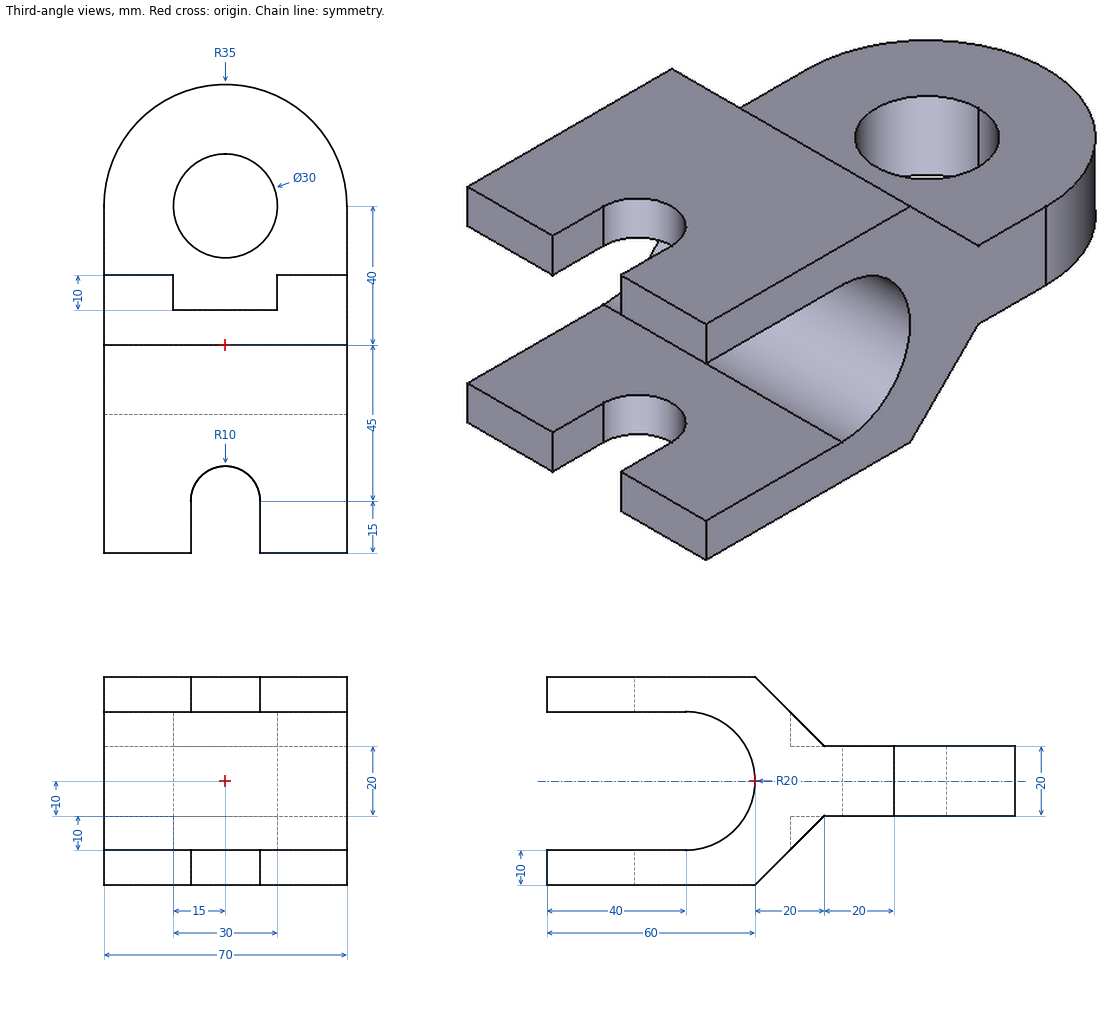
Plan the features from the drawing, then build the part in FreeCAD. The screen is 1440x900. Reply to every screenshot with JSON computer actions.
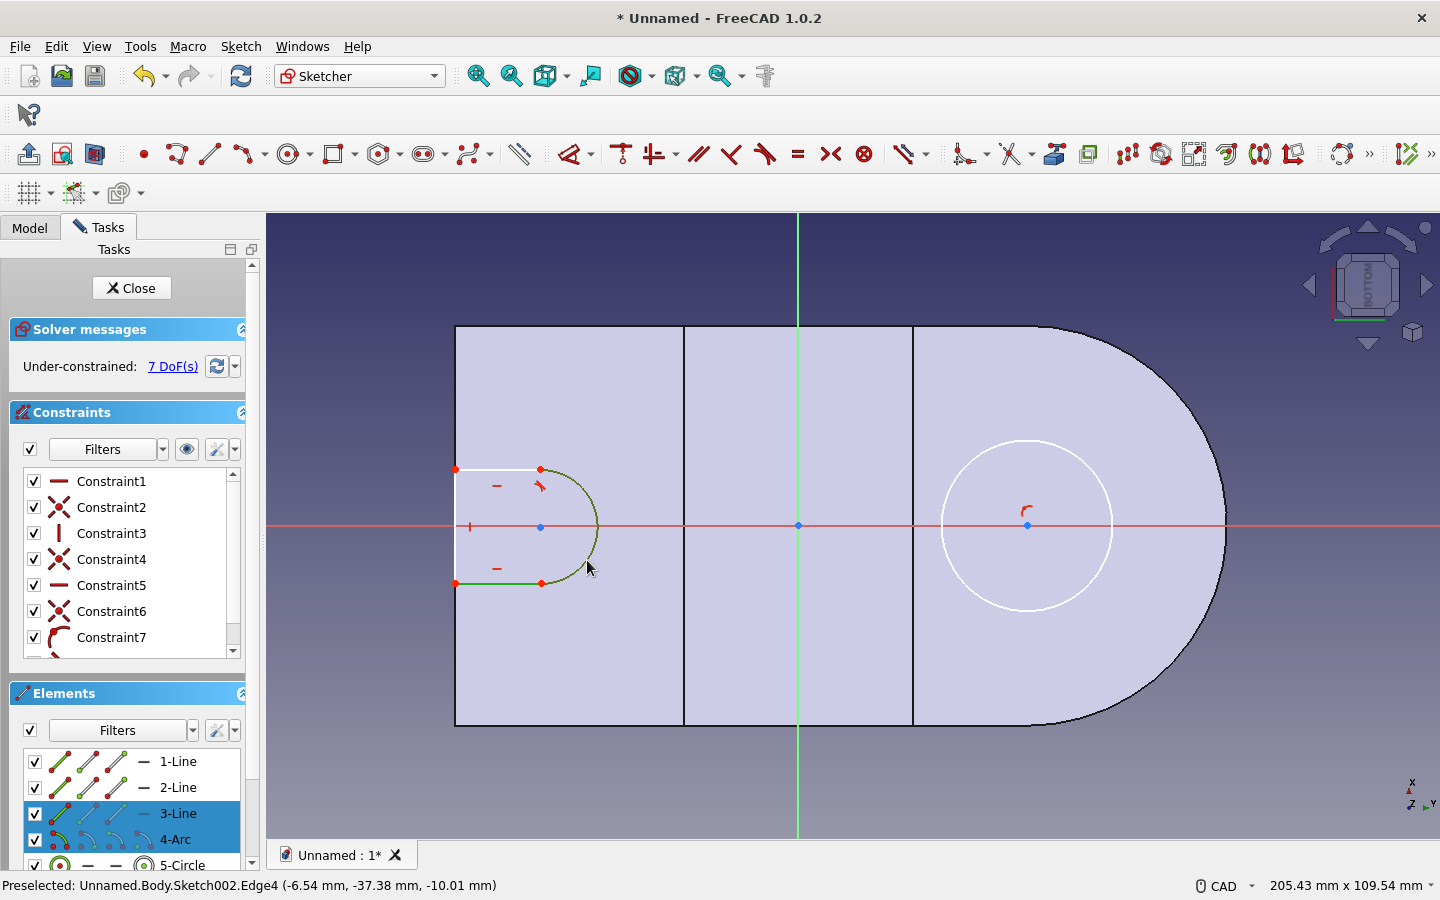
{"action": "key", "text": "t"}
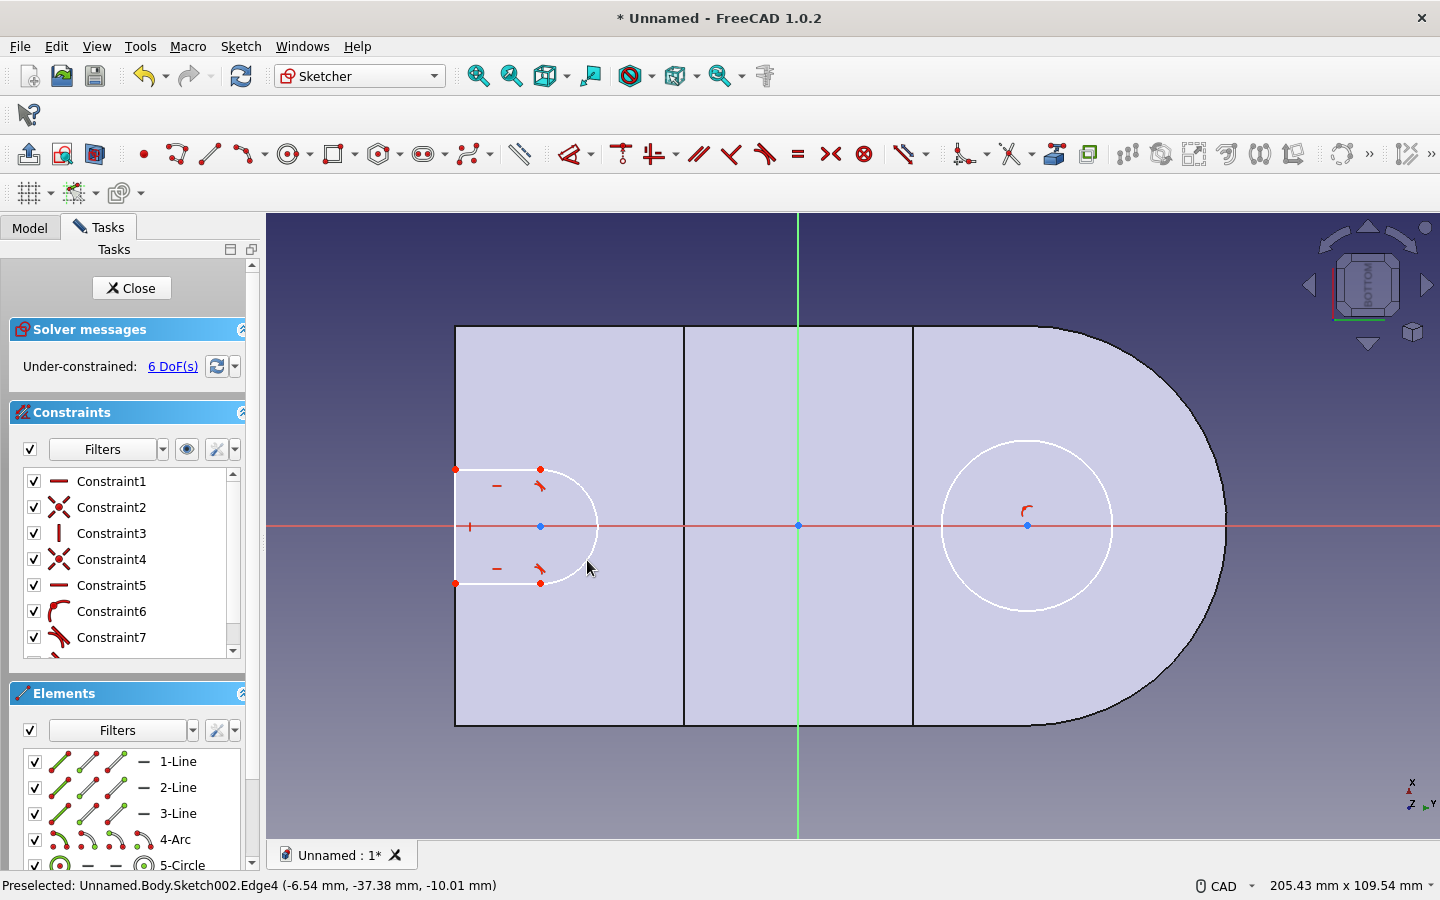
{"action": "left_click", "coordinate": [541, 527]}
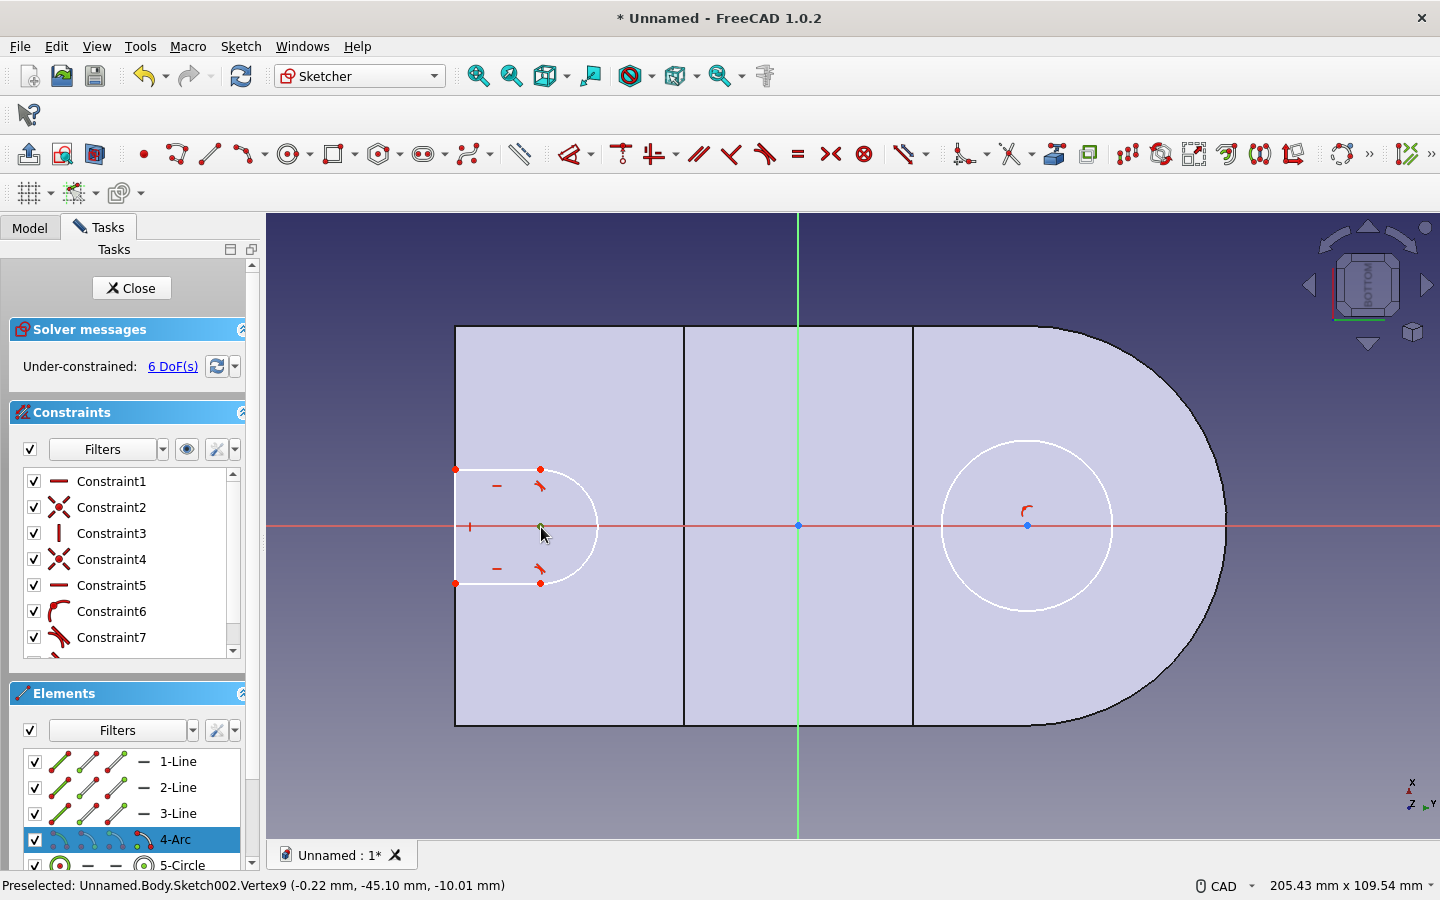
{"action": "left_click", "coordinate": [364, 526]}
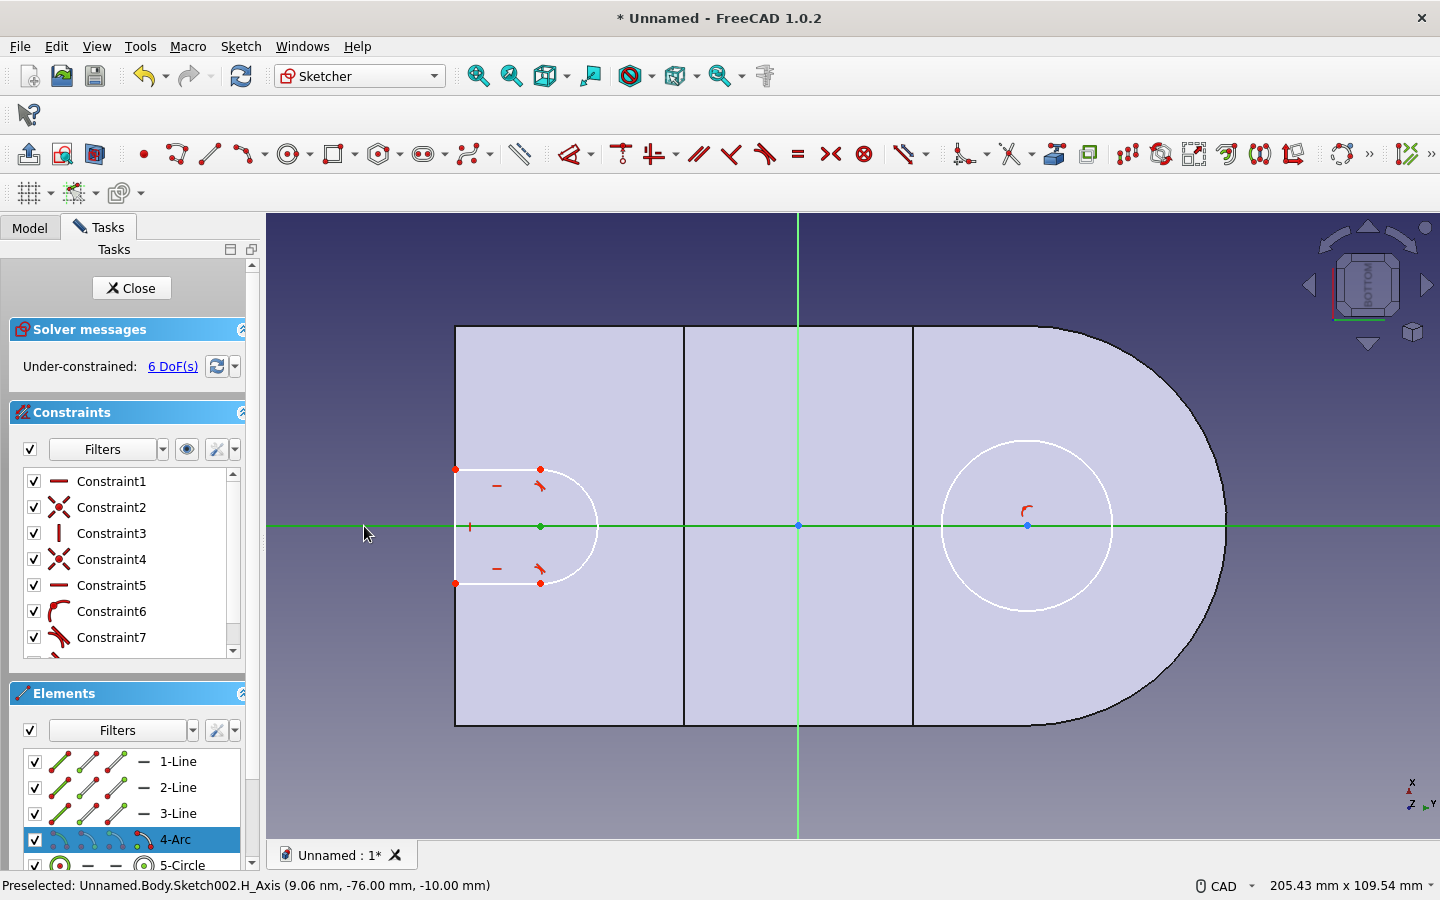
{"action": "key", "text": "c"}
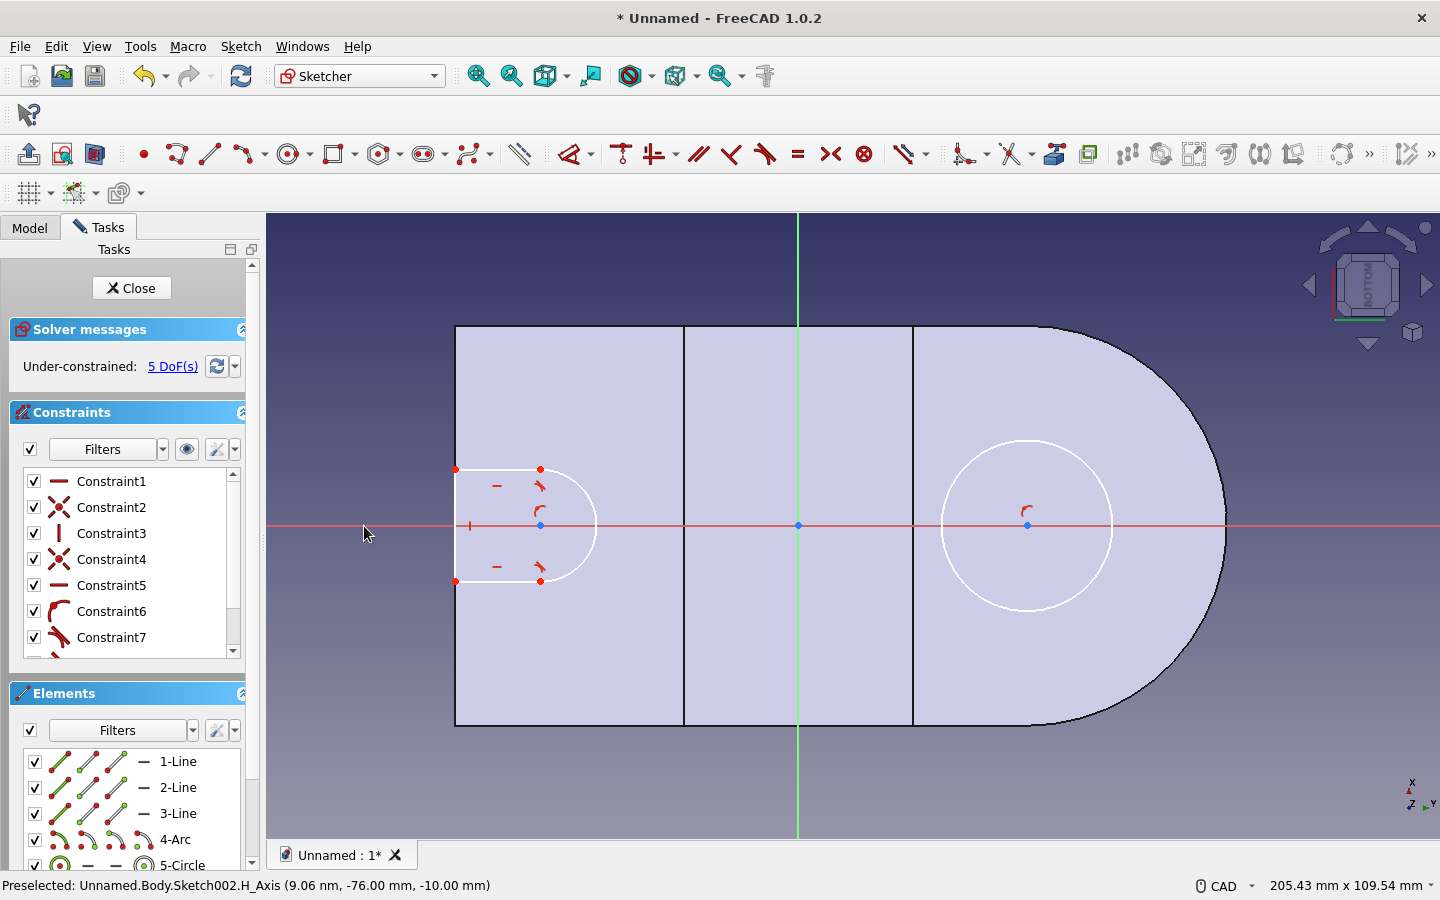
{"action": "key", "text": "d"}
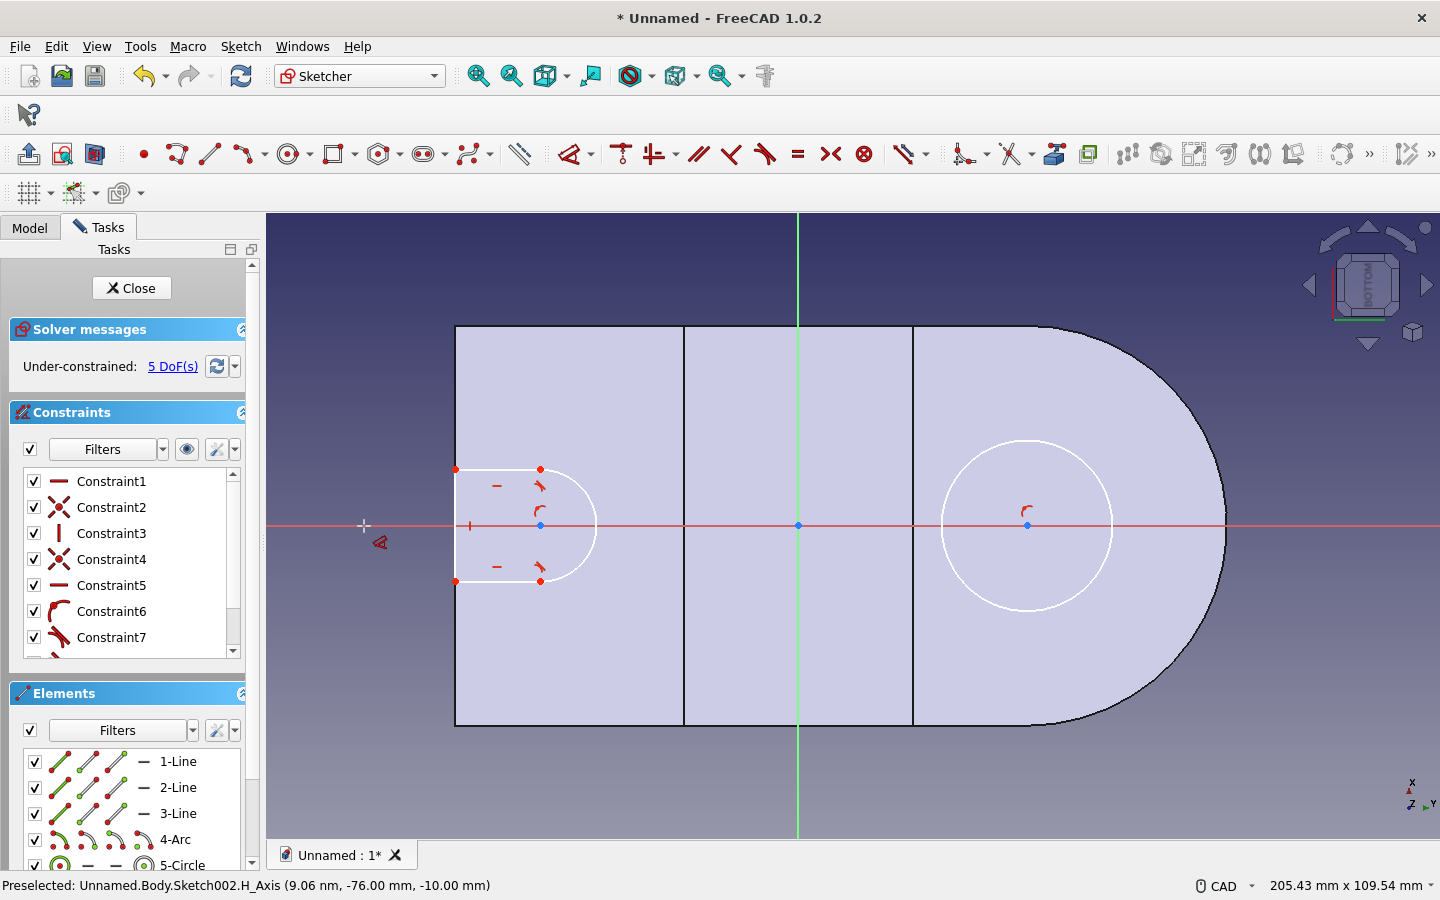
{"action": "left_click", "coordinate": [586, 559]}
{"action": "left_click", "coordinate": [612, 578]}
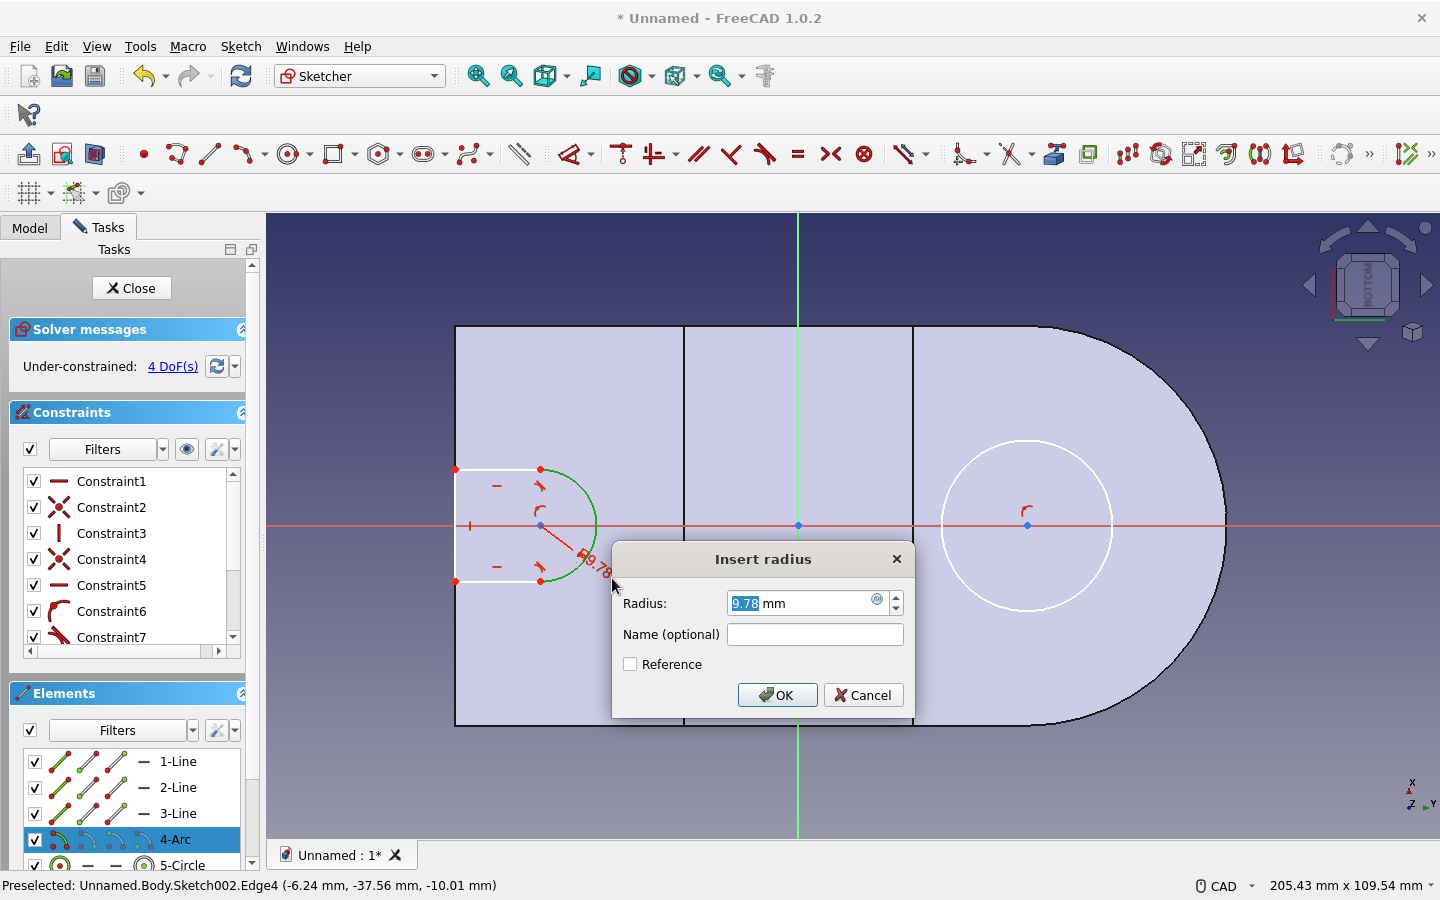
{"action": "type", "text": "10"}
{"action": "key", "text": "Return"}